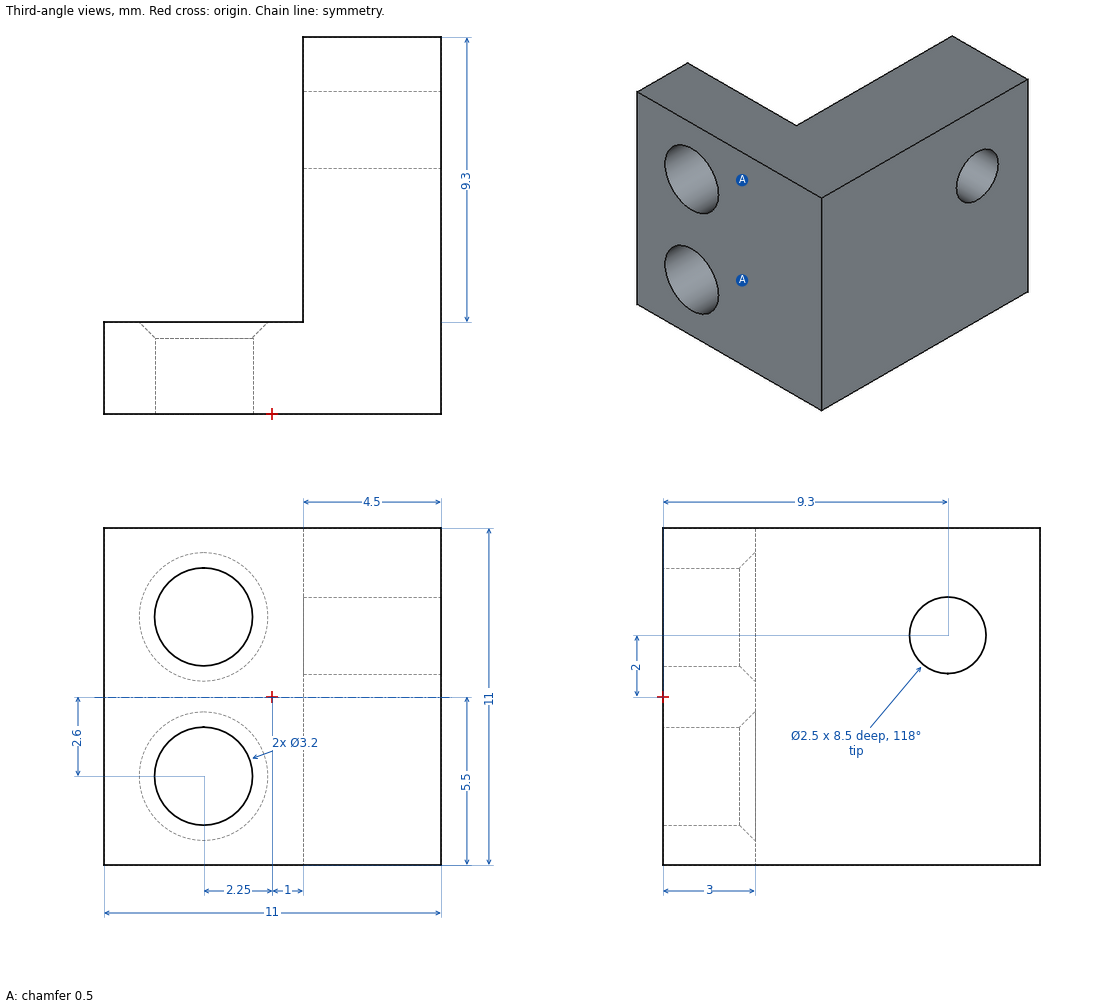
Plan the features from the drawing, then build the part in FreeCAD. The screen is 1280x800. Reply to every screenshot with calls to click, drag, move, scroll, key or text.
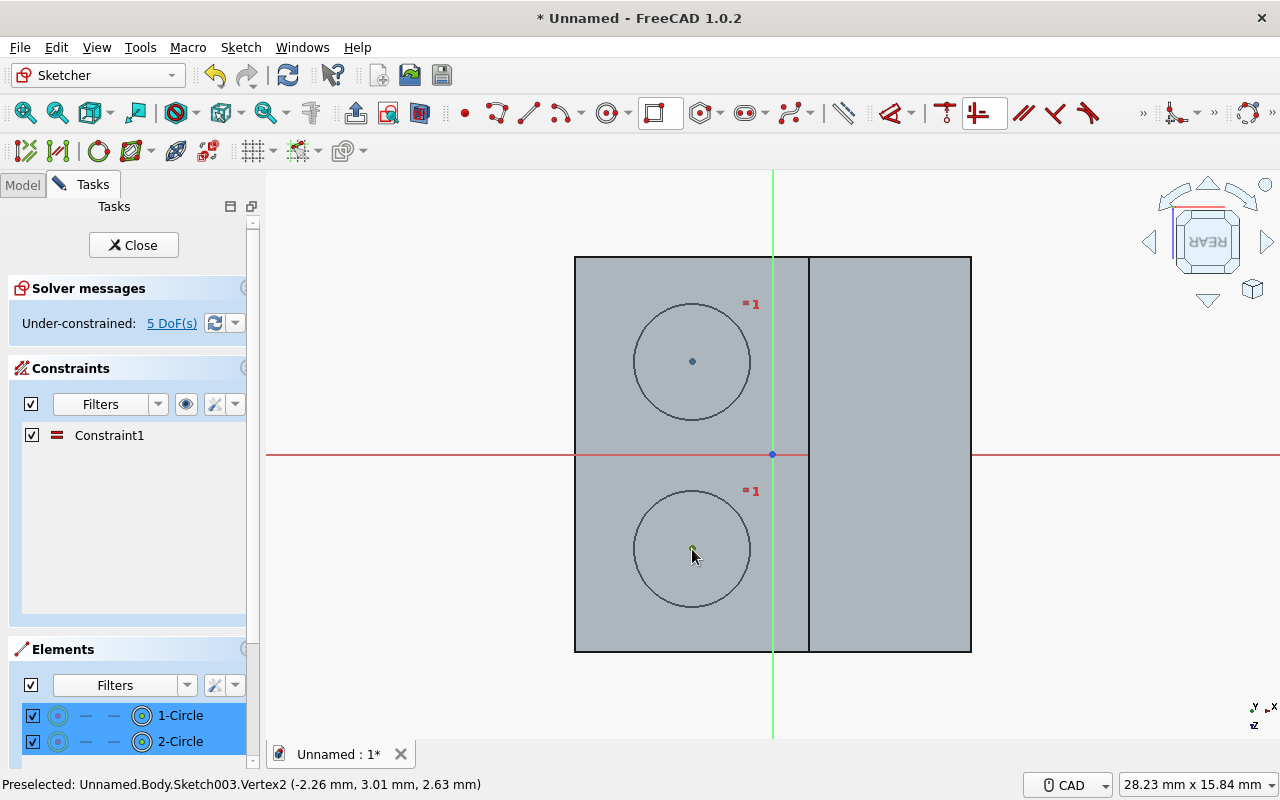
click(353, 454)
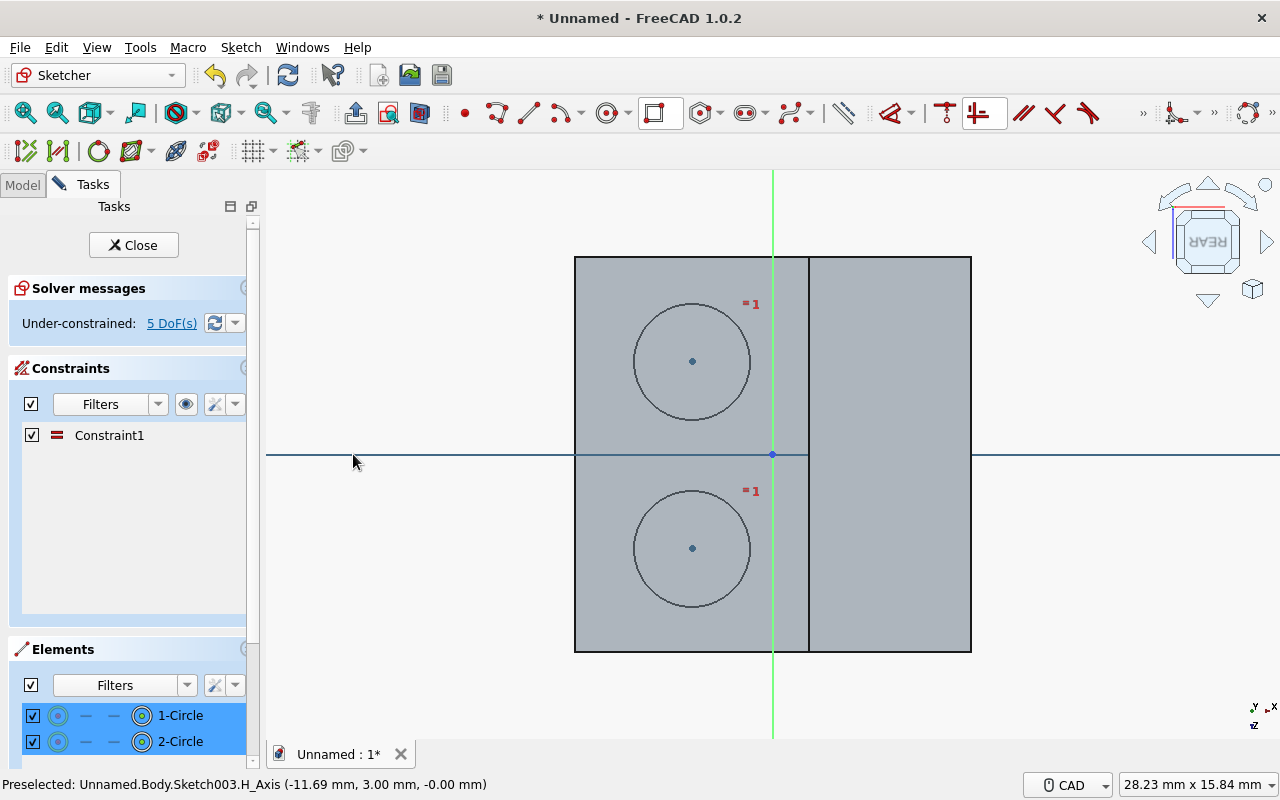
key(s)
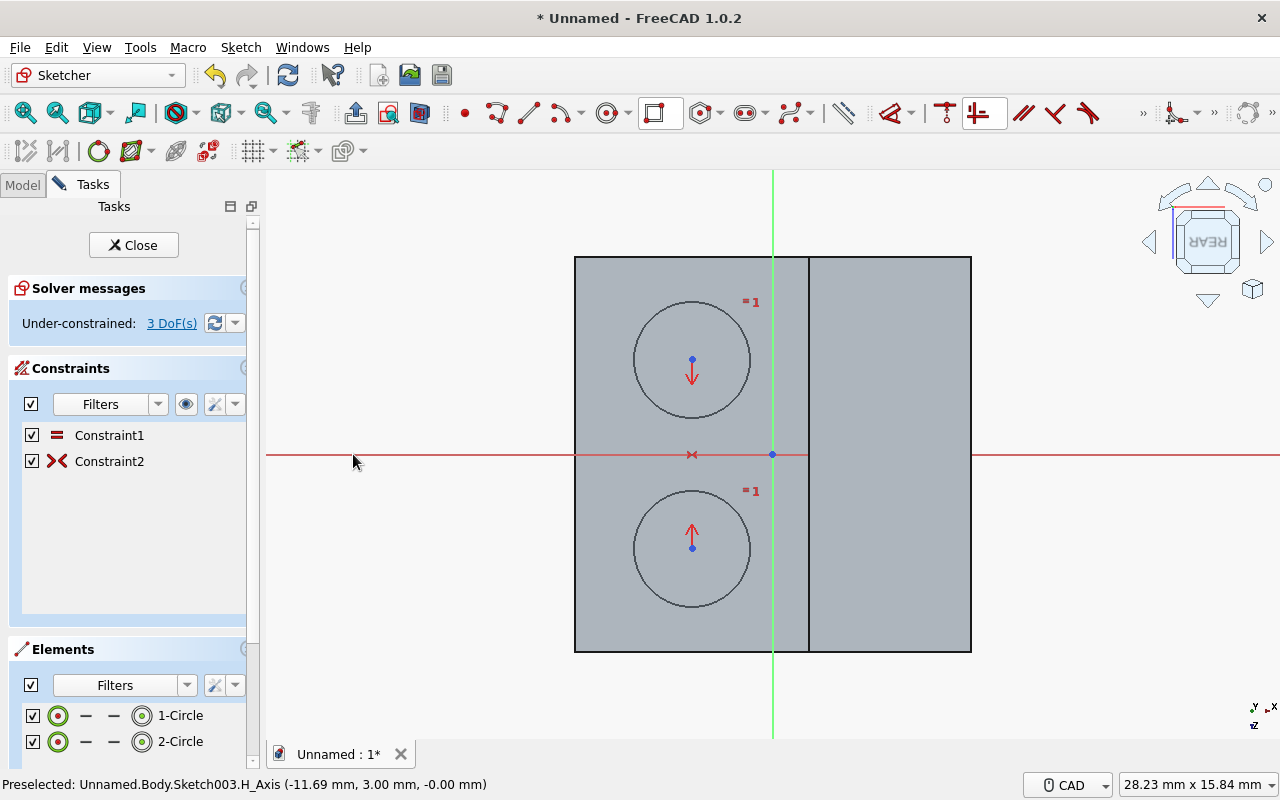
click(890, 114)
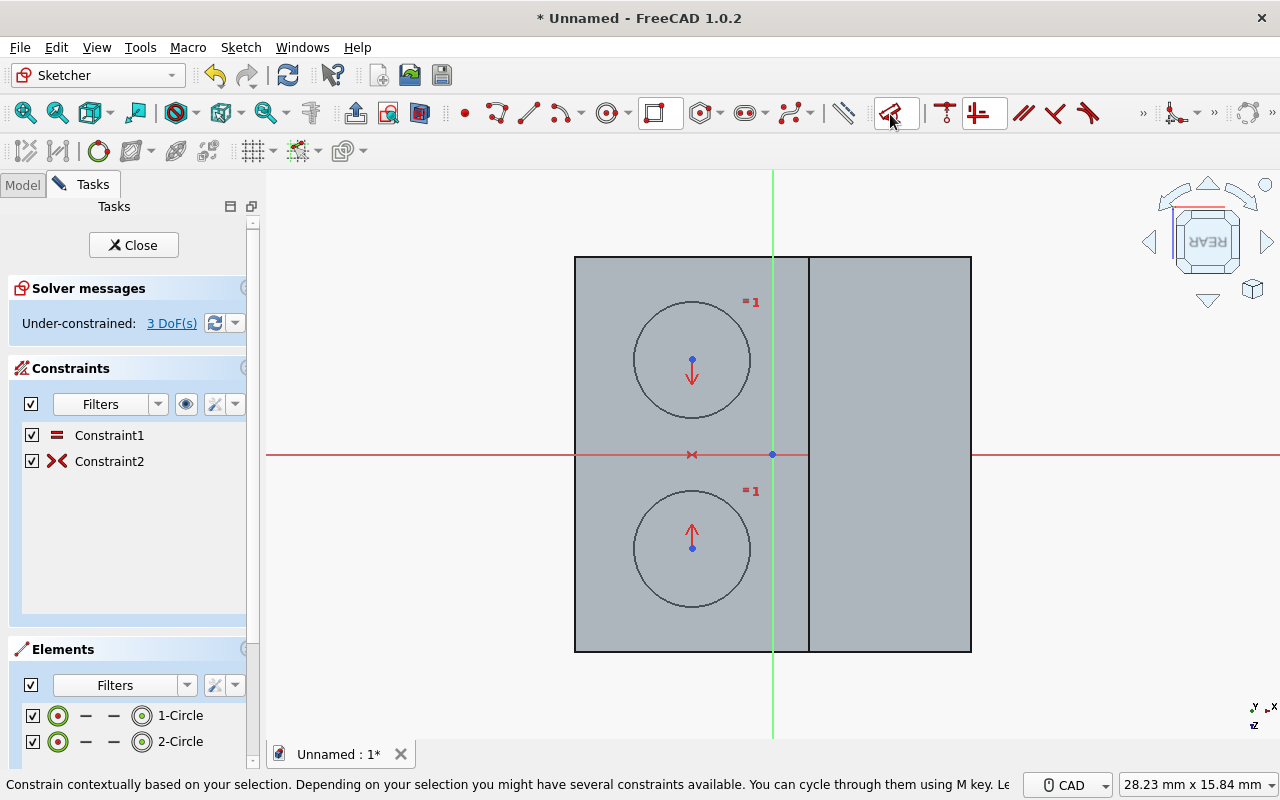
click(733, 319)
click(756, 296)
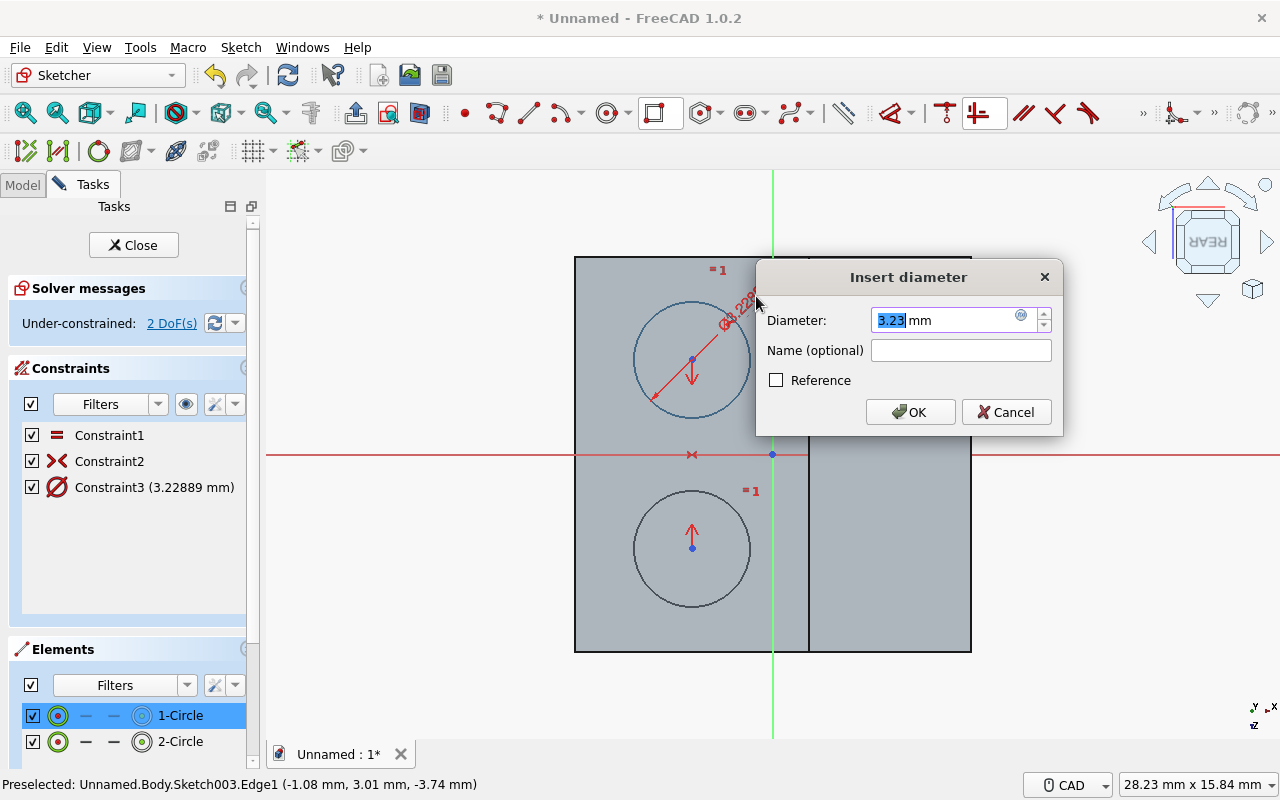
text(3.2)
key(Return)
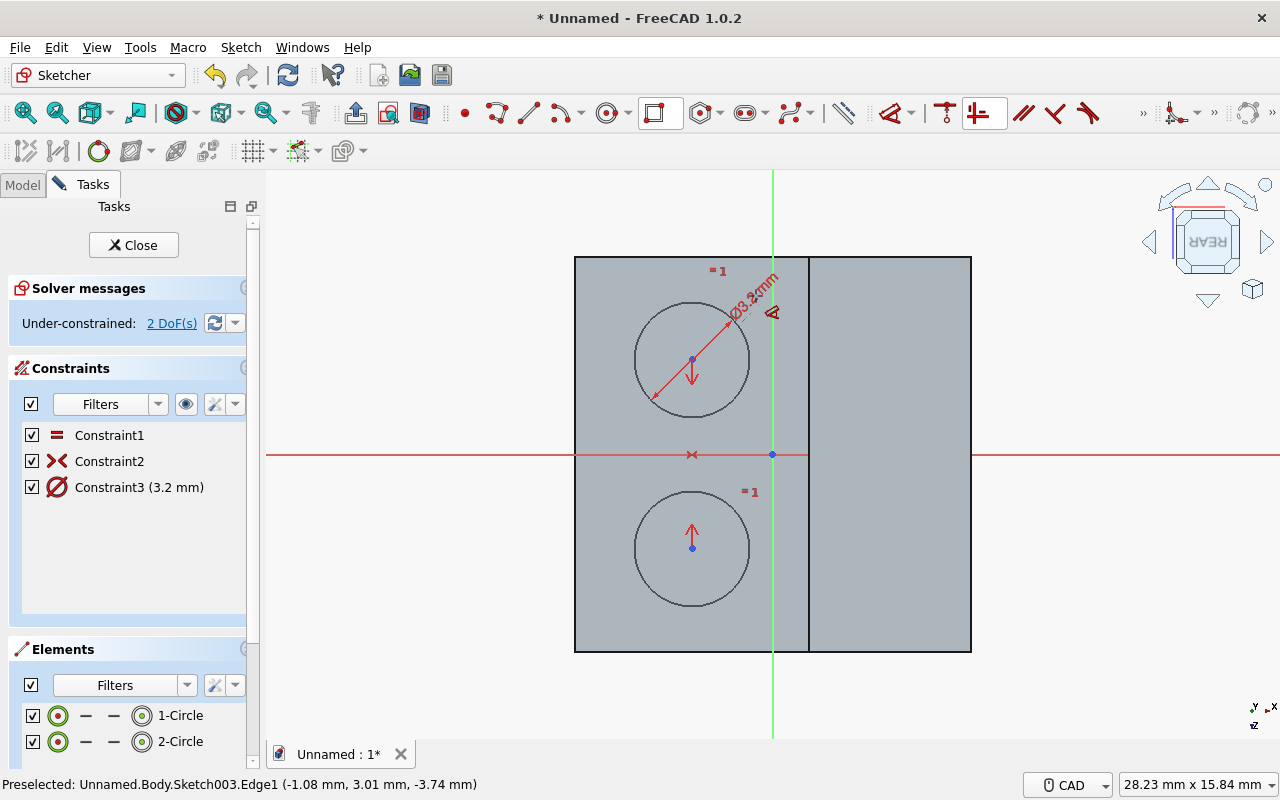
click(692, 360)
click(807, 407)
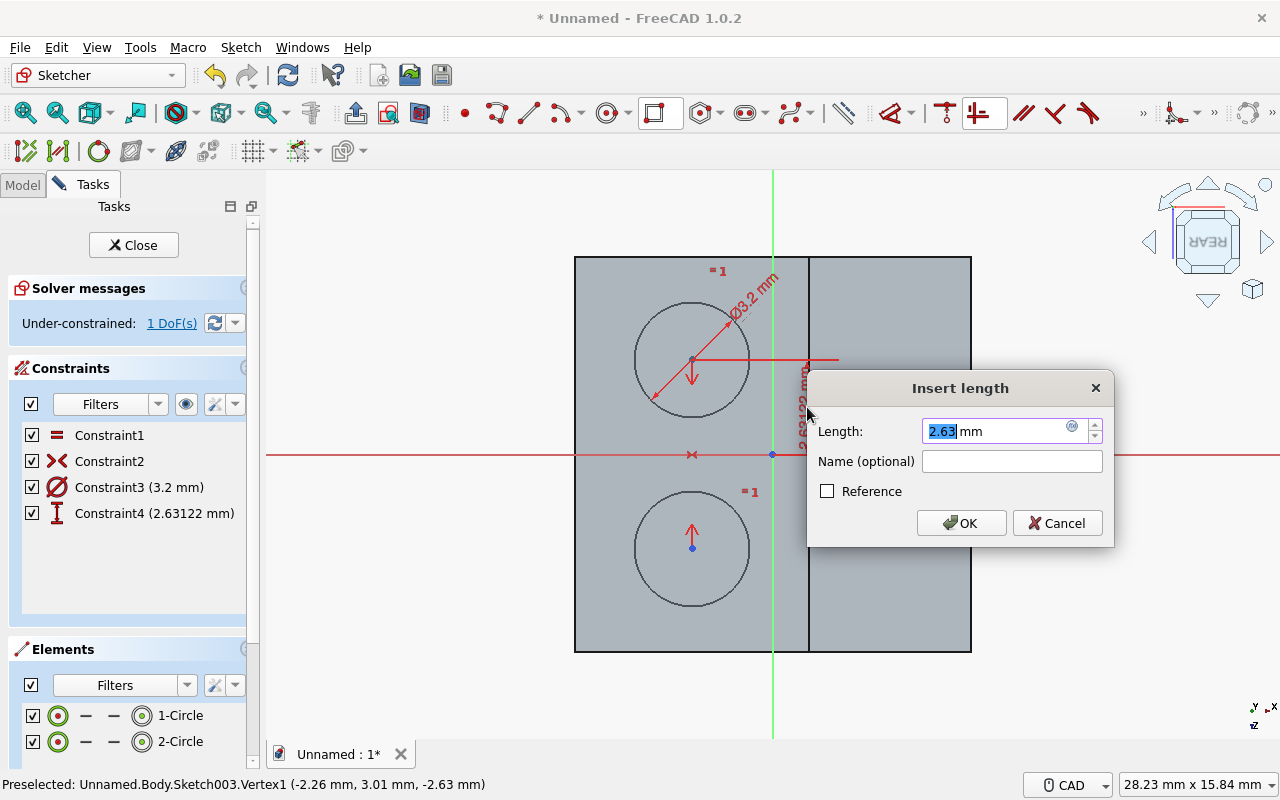
text(2.6)
key(Return)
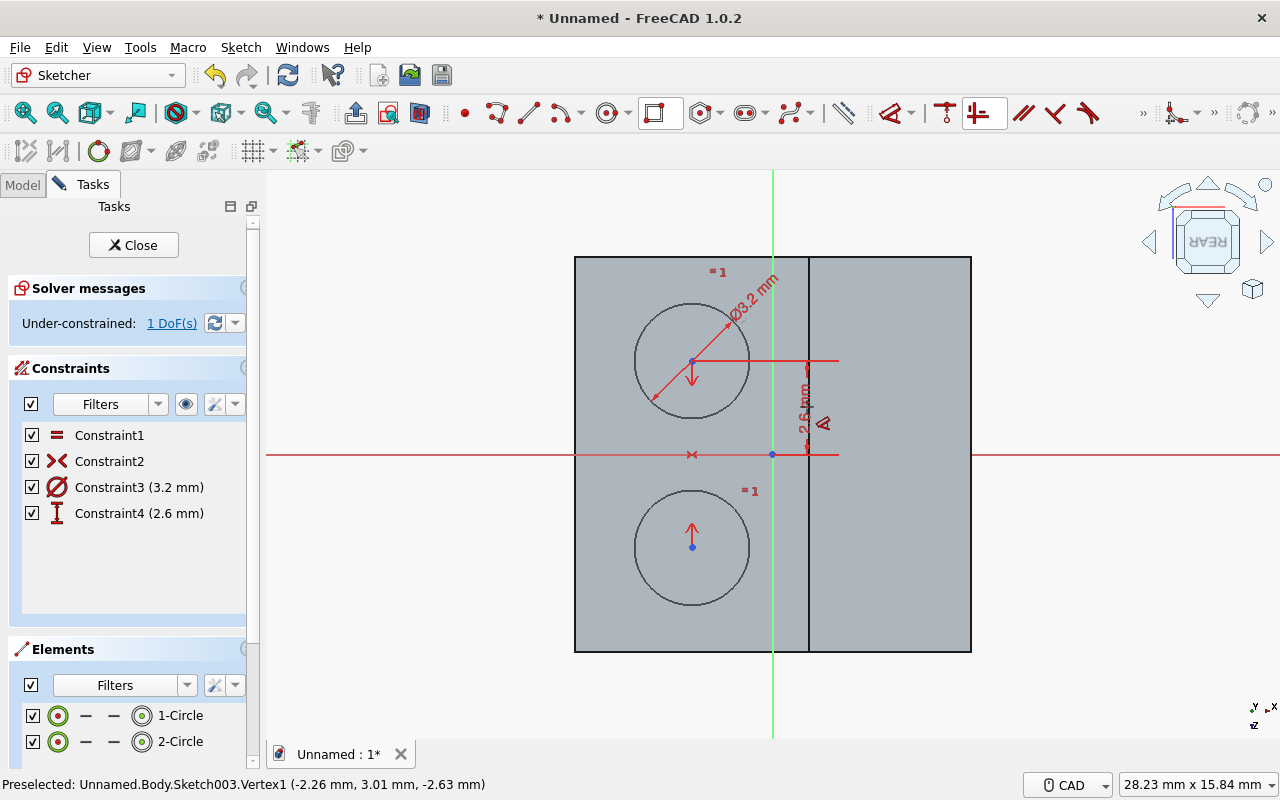
click(692, 361)
click(714, 327)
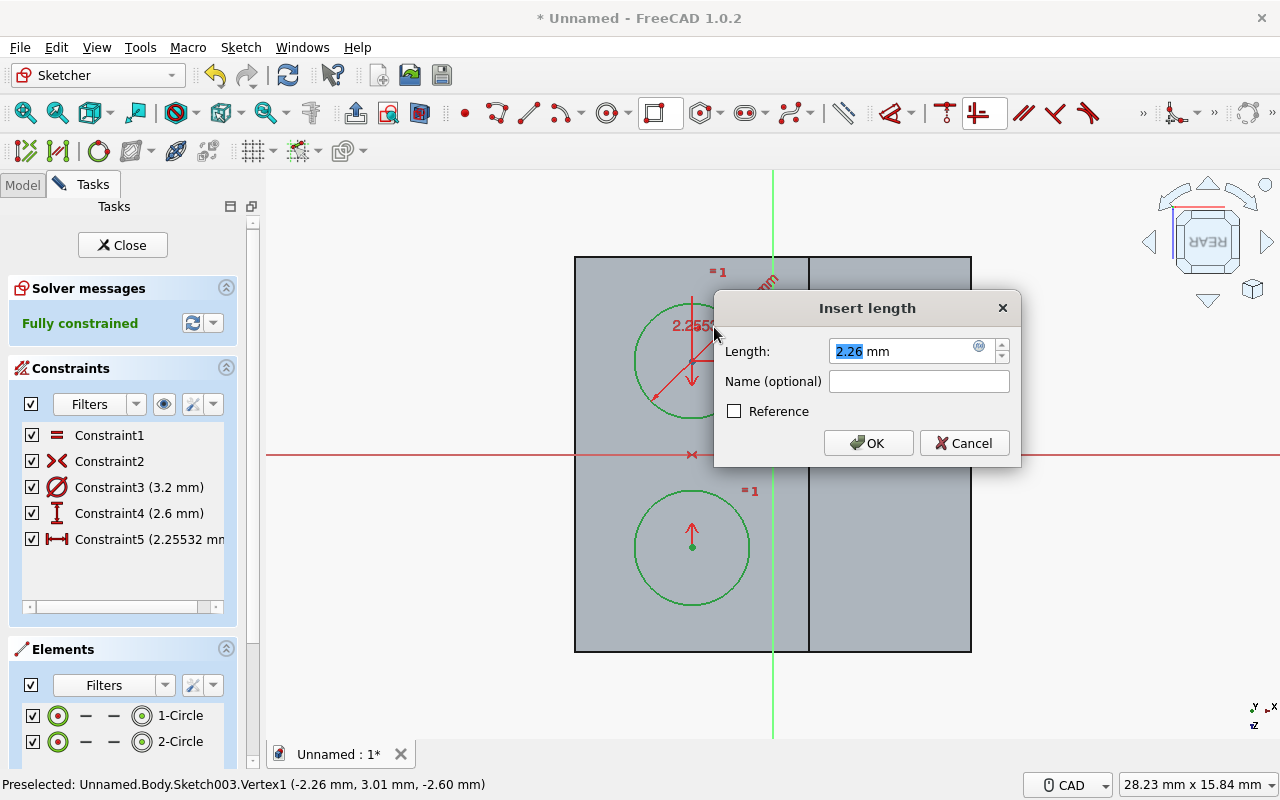
text(2.25)
key(Return)
key(Escape)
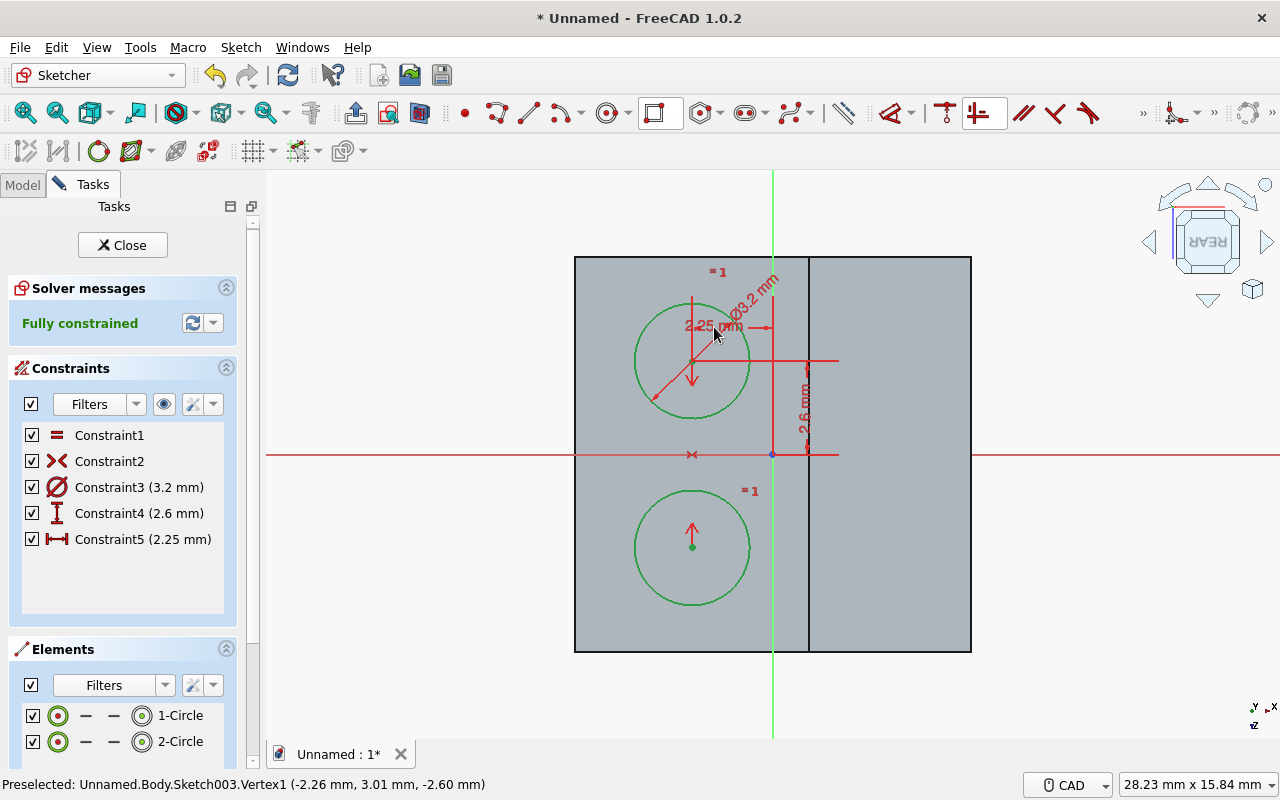
click(123, 245)